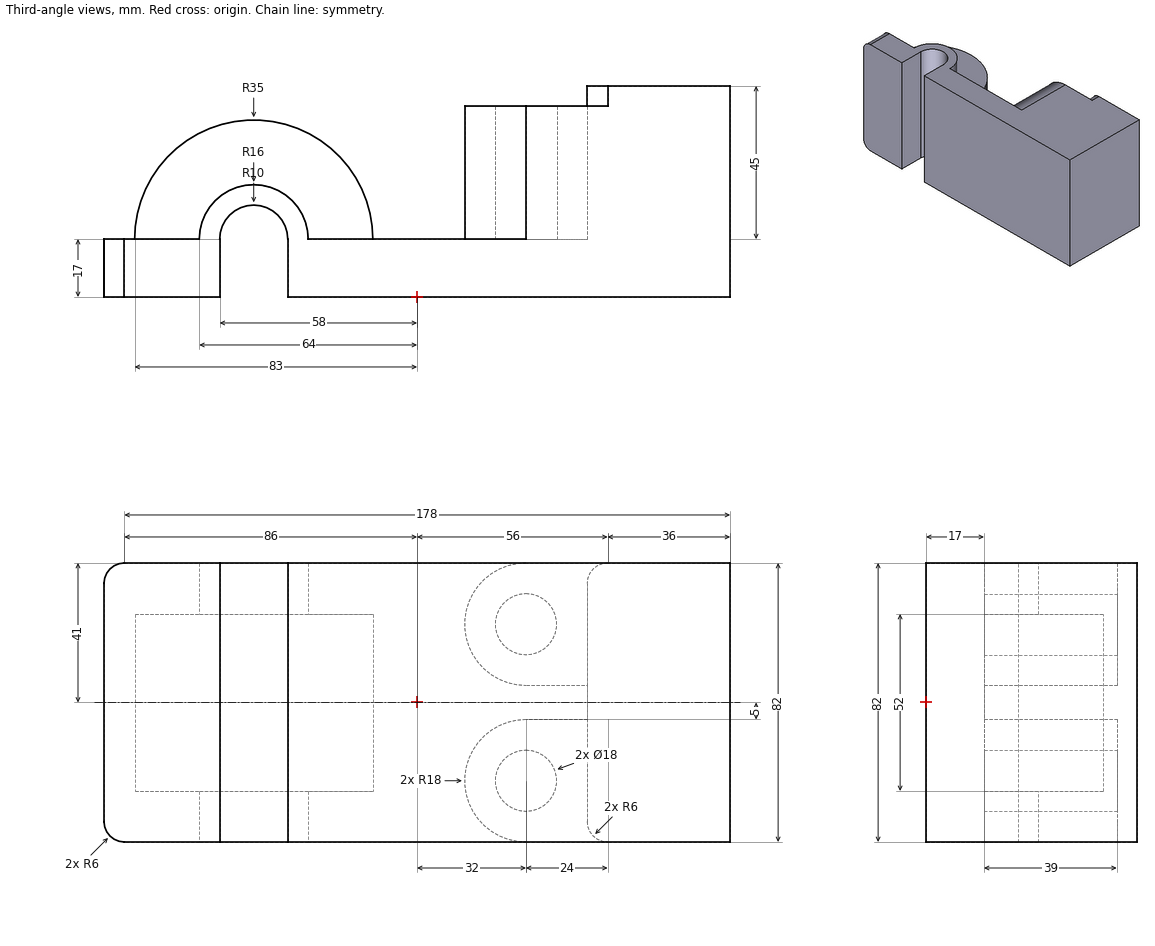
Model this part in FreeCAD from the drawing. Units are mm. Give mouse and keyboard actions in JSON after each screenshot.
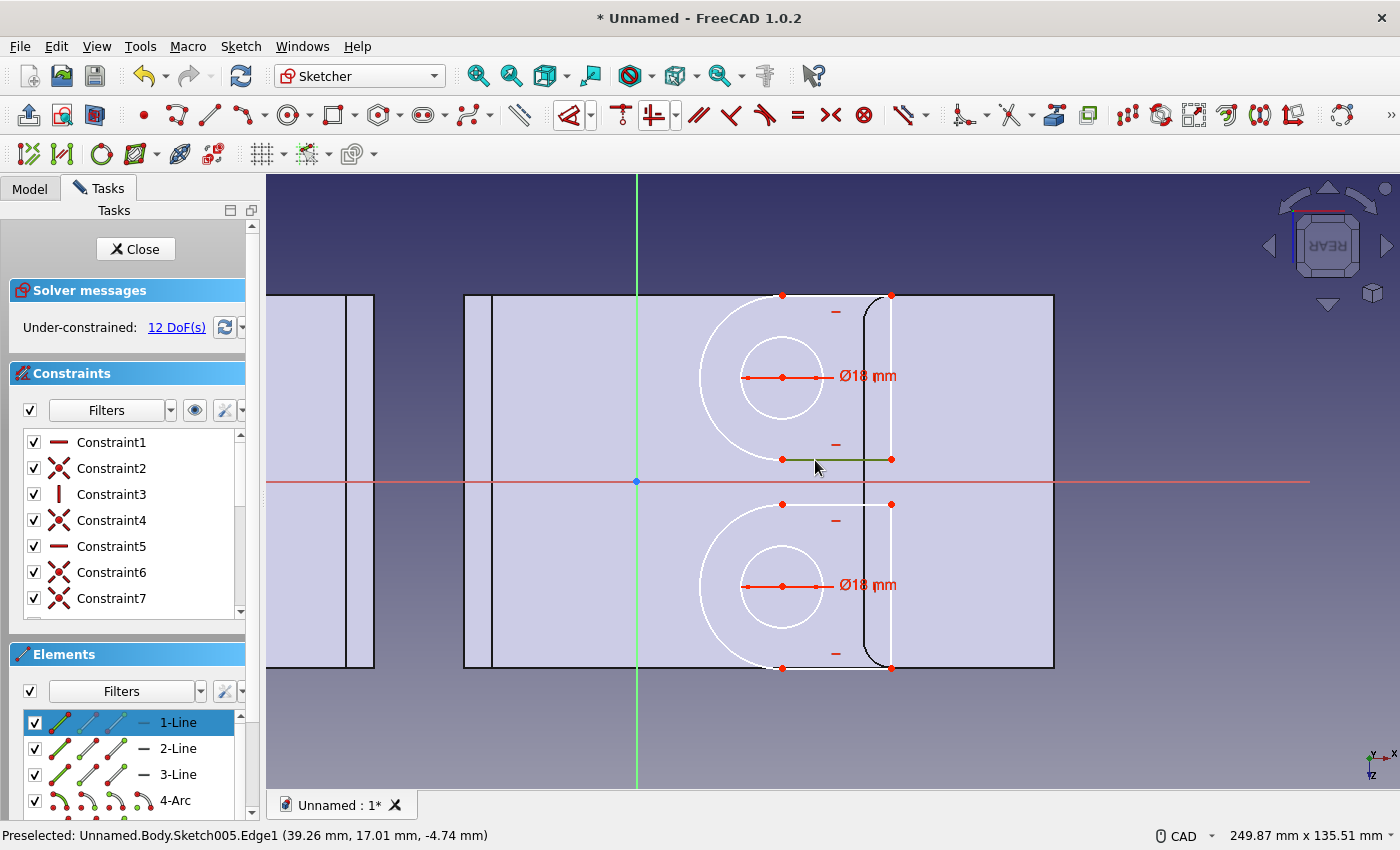
{"action": "left_click", "coordinate": [716, 330]}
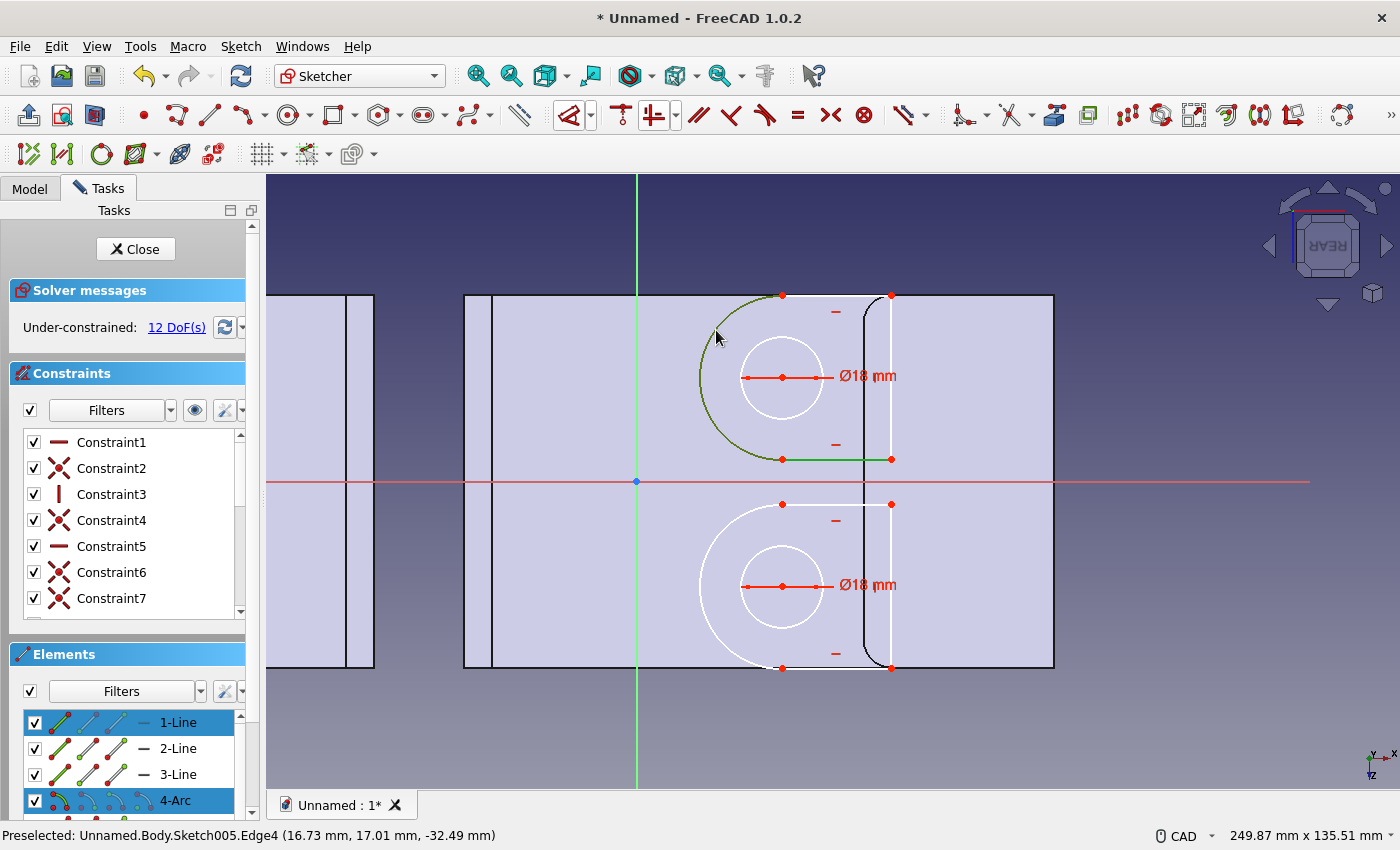
{"action": "left_click", "coordinate": [765, 116]}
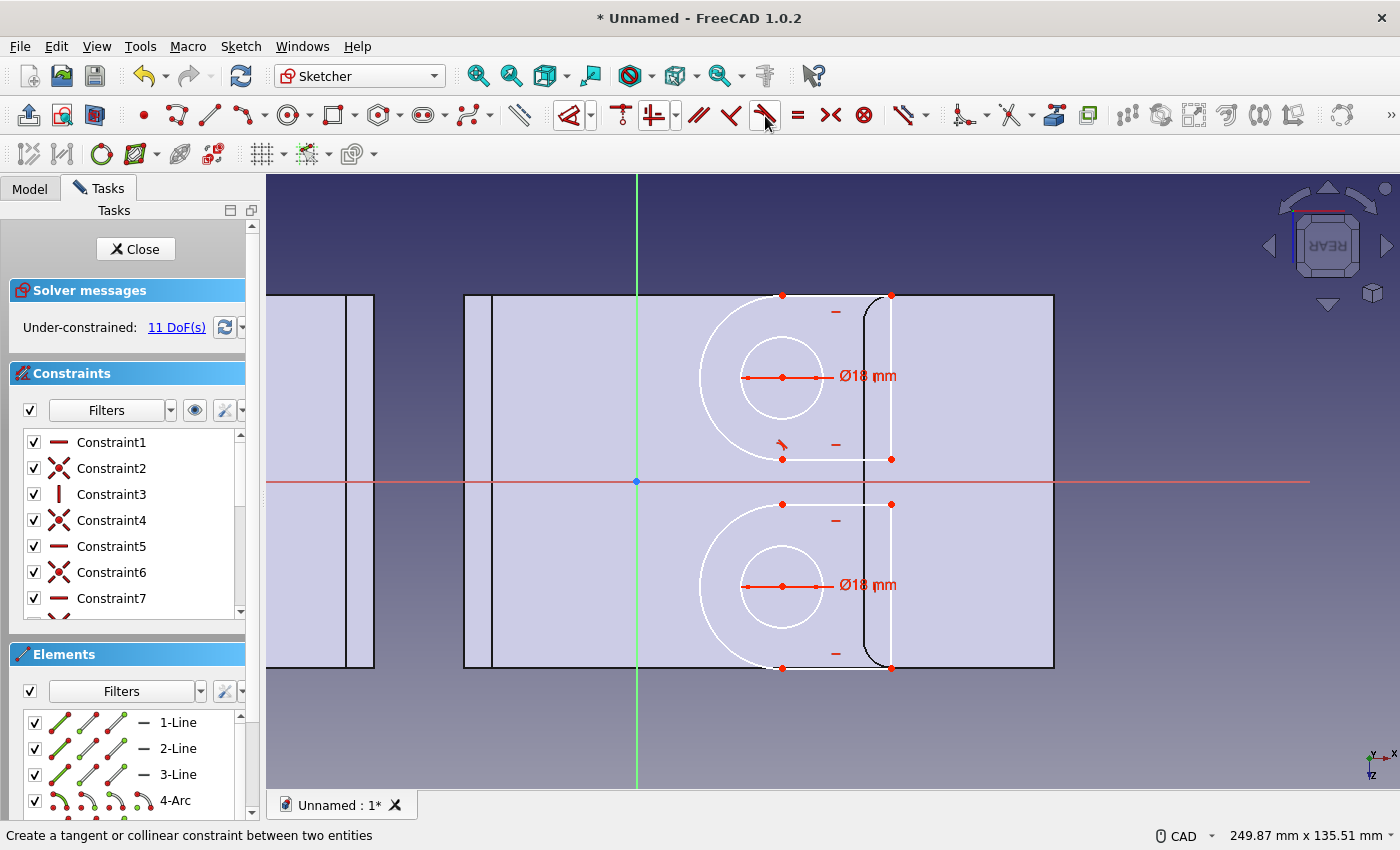
{"action": "left_click", "coordinate": [858, 296]}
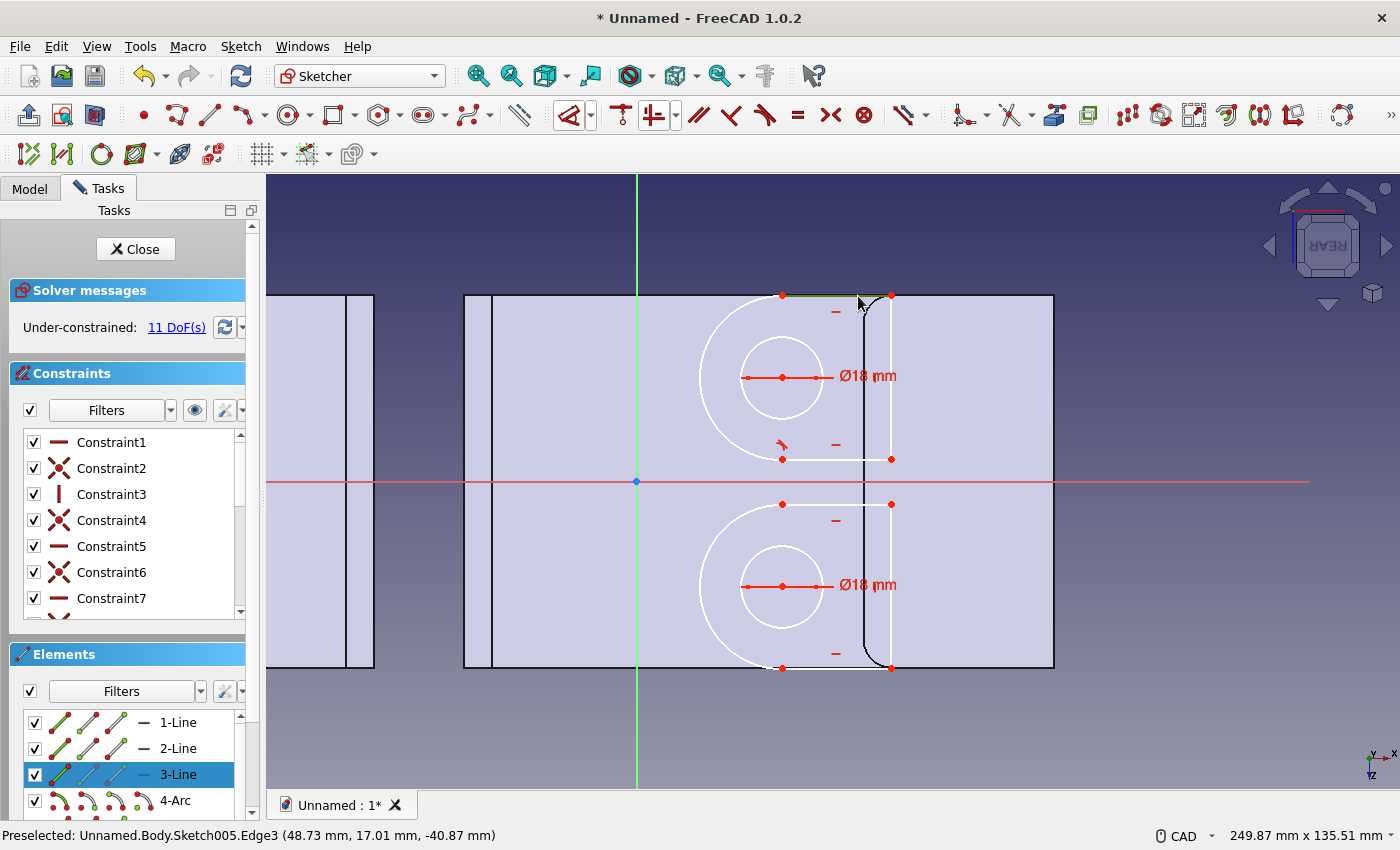
{"action": "left_click", "coordinate": [716, 330]}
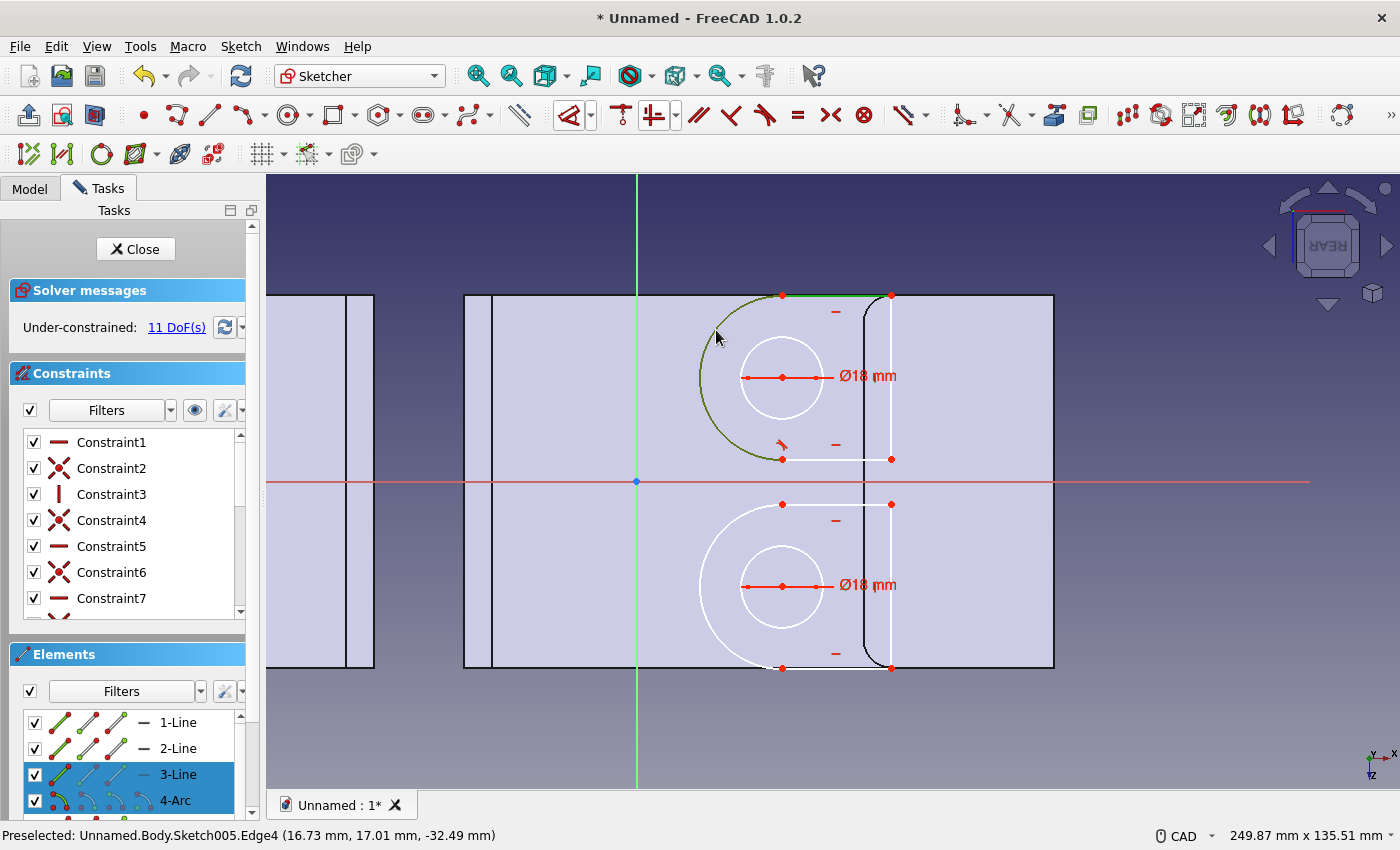
{"action": "left_click", "coordinate": [765, 116]}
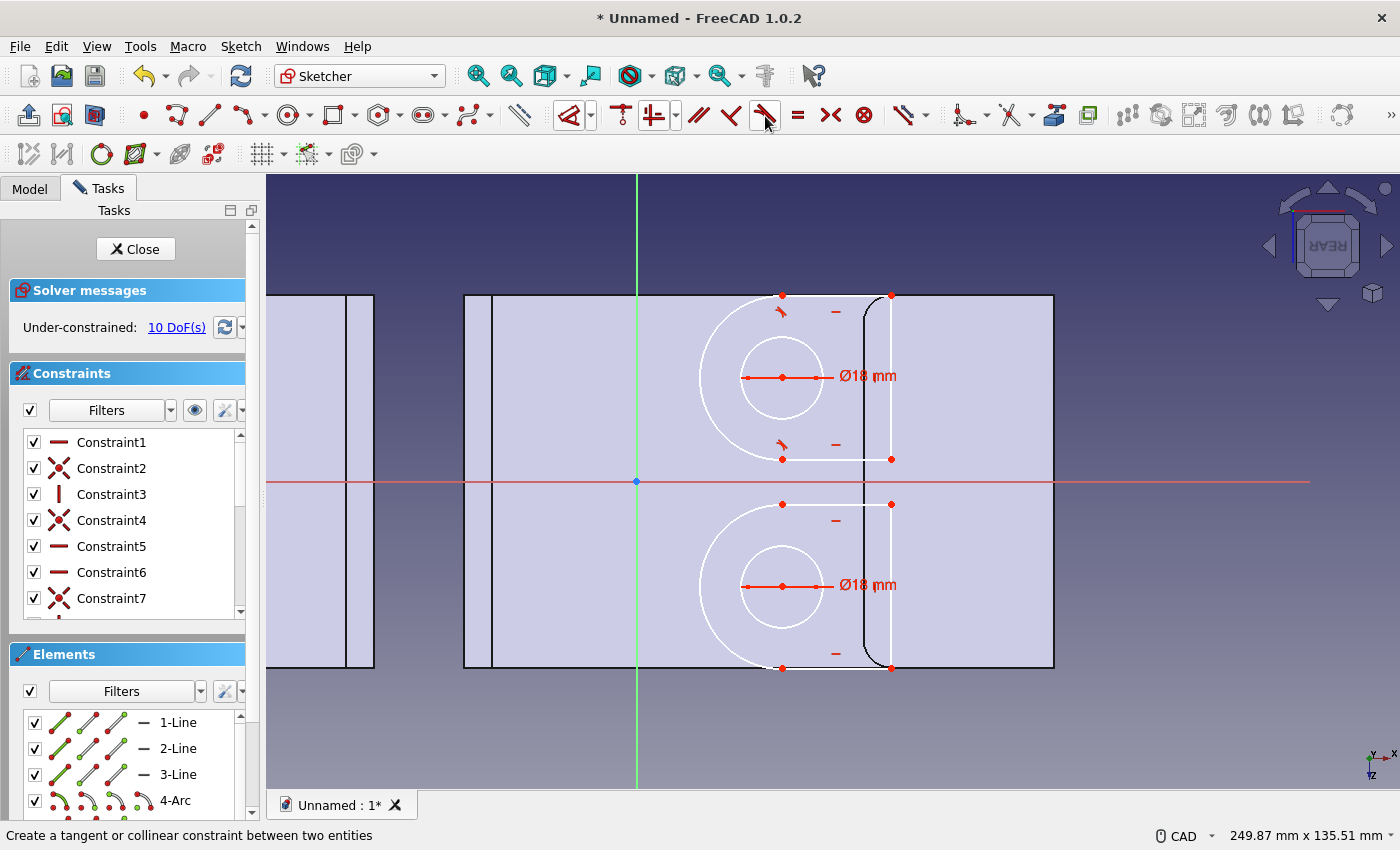
{"action": "left_click", "coordinate": [815, 669]}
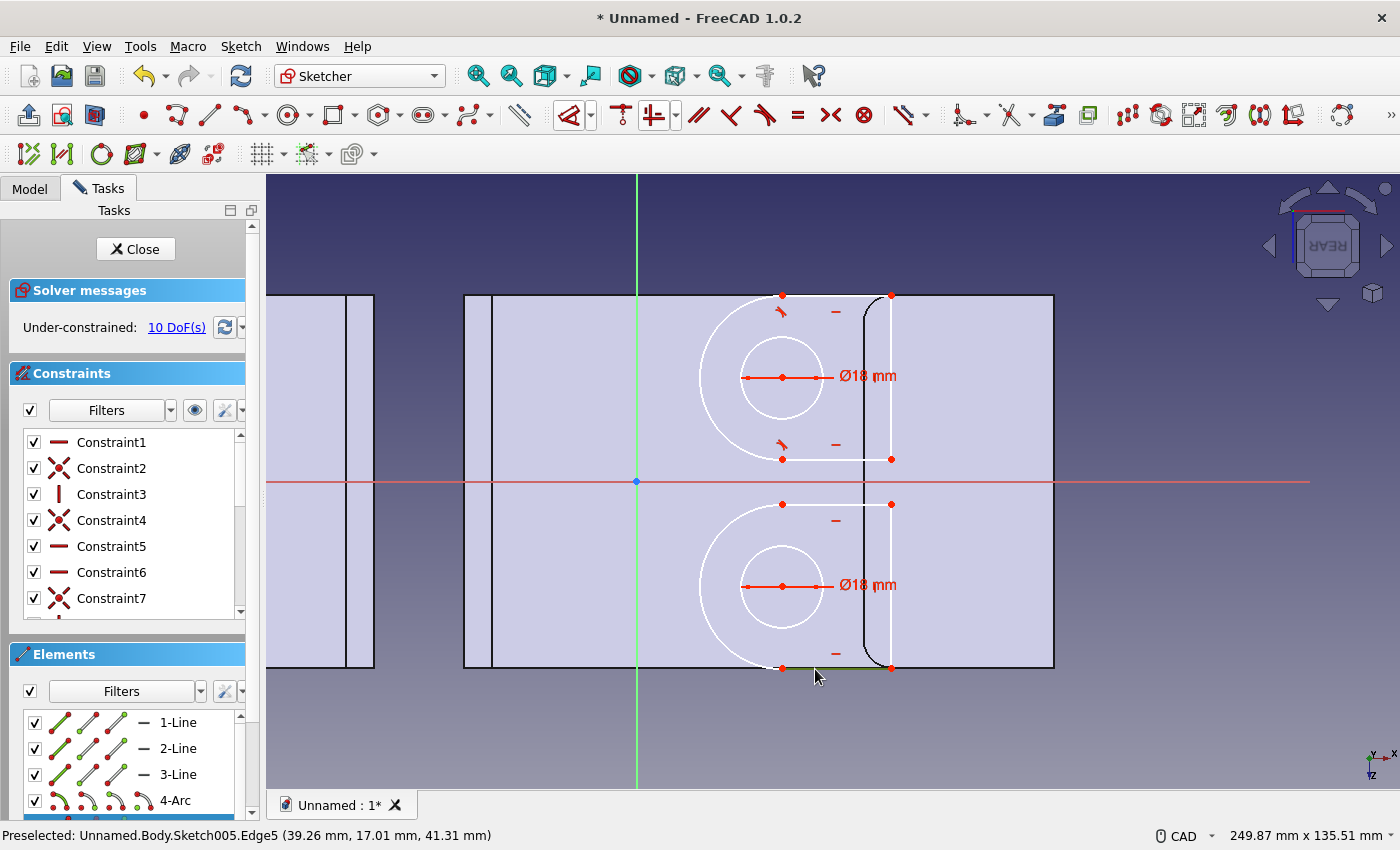
{"action": "left_click", "coordinate": [716, 539]}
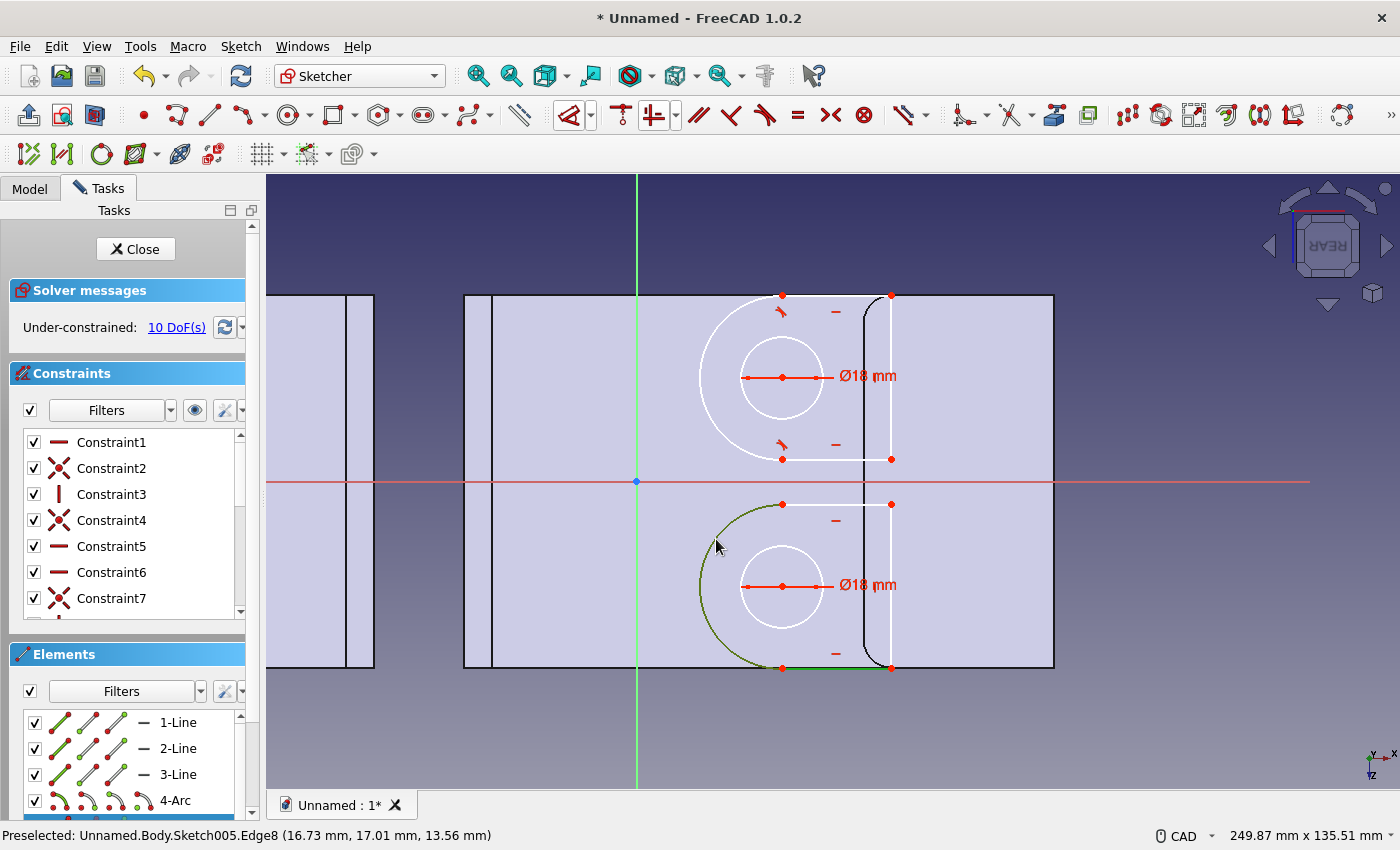
{"action": "left_click", "coordinate": [765, 116]}